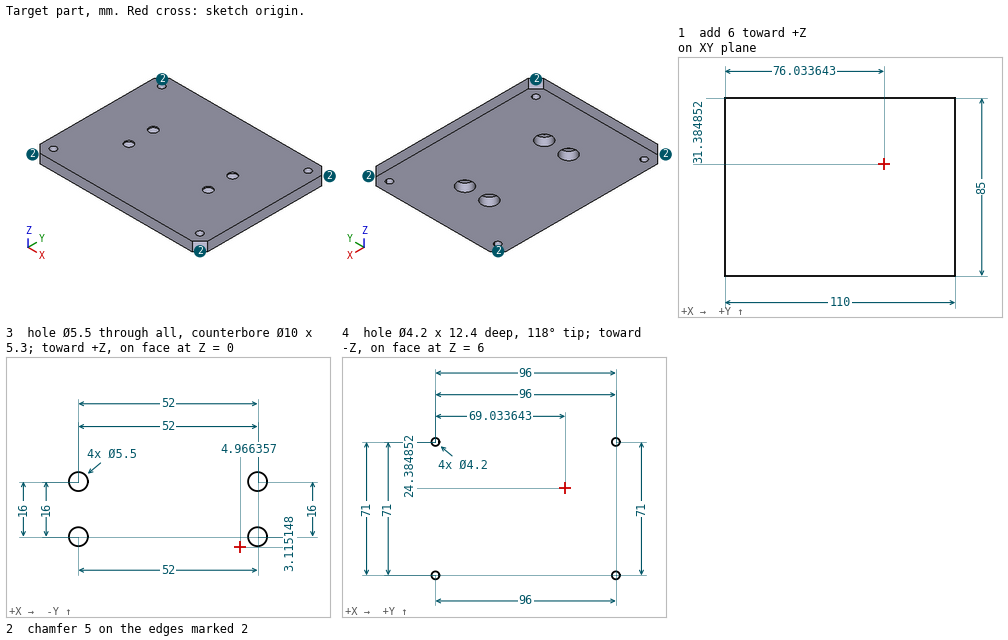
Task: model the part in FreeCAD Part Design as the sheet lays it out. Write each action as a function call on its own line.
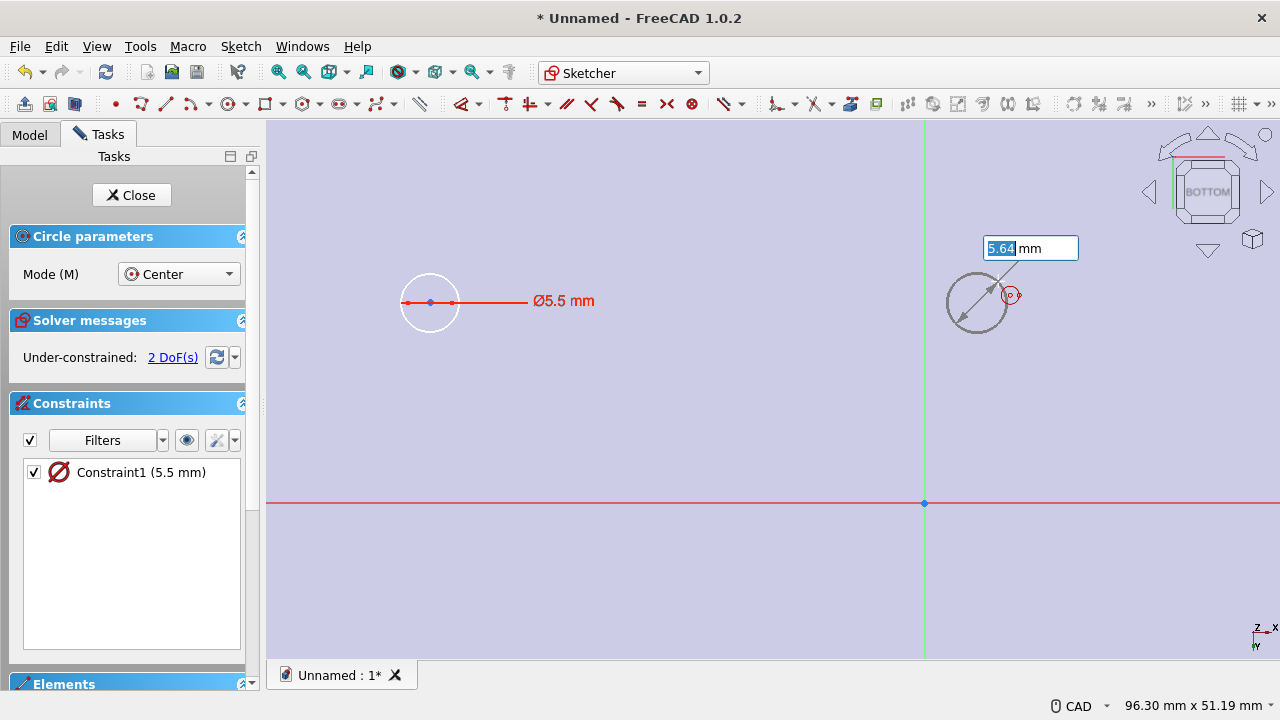
text(5.5)
key(Return)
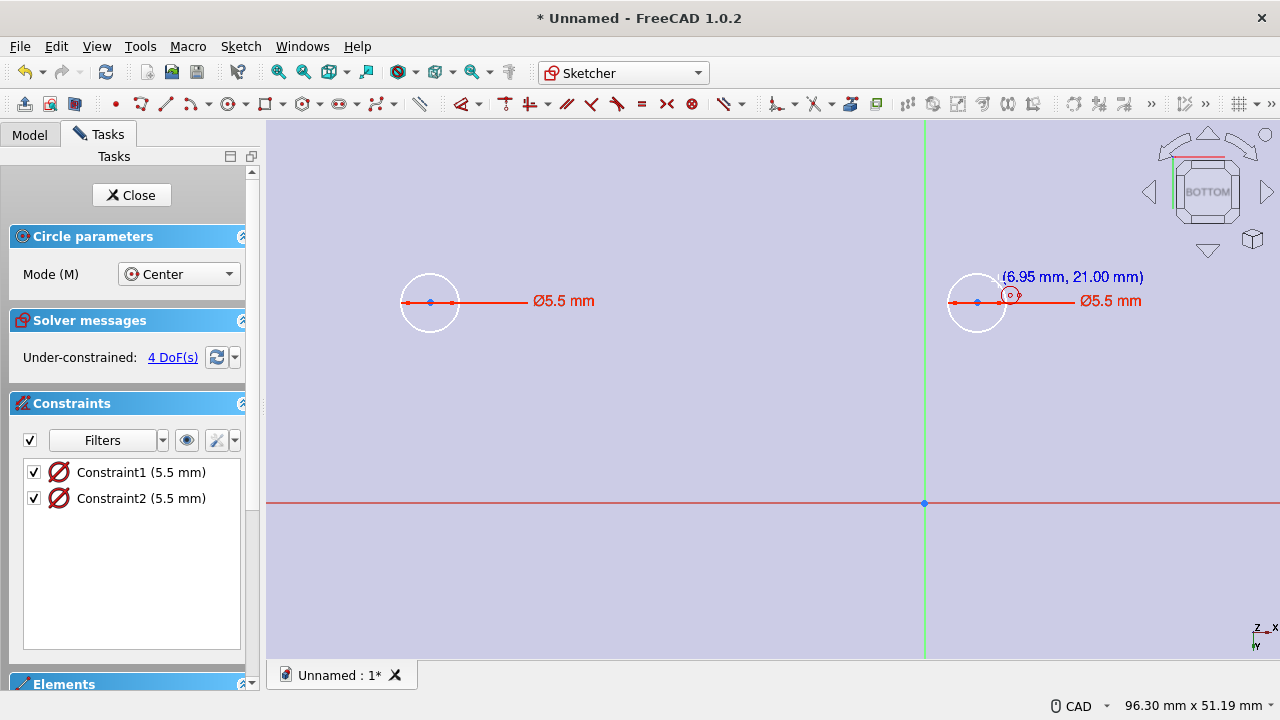
click(977, 470)
move(998, 450)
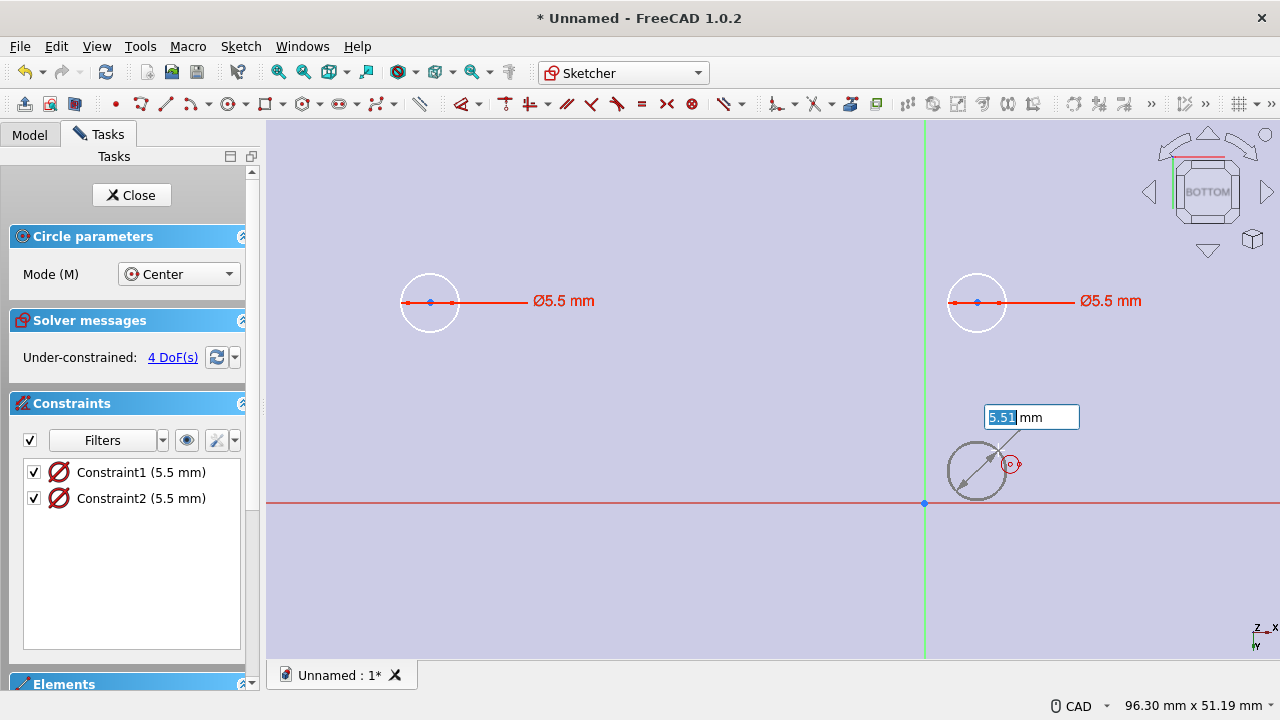
text(5.5)
key(Return)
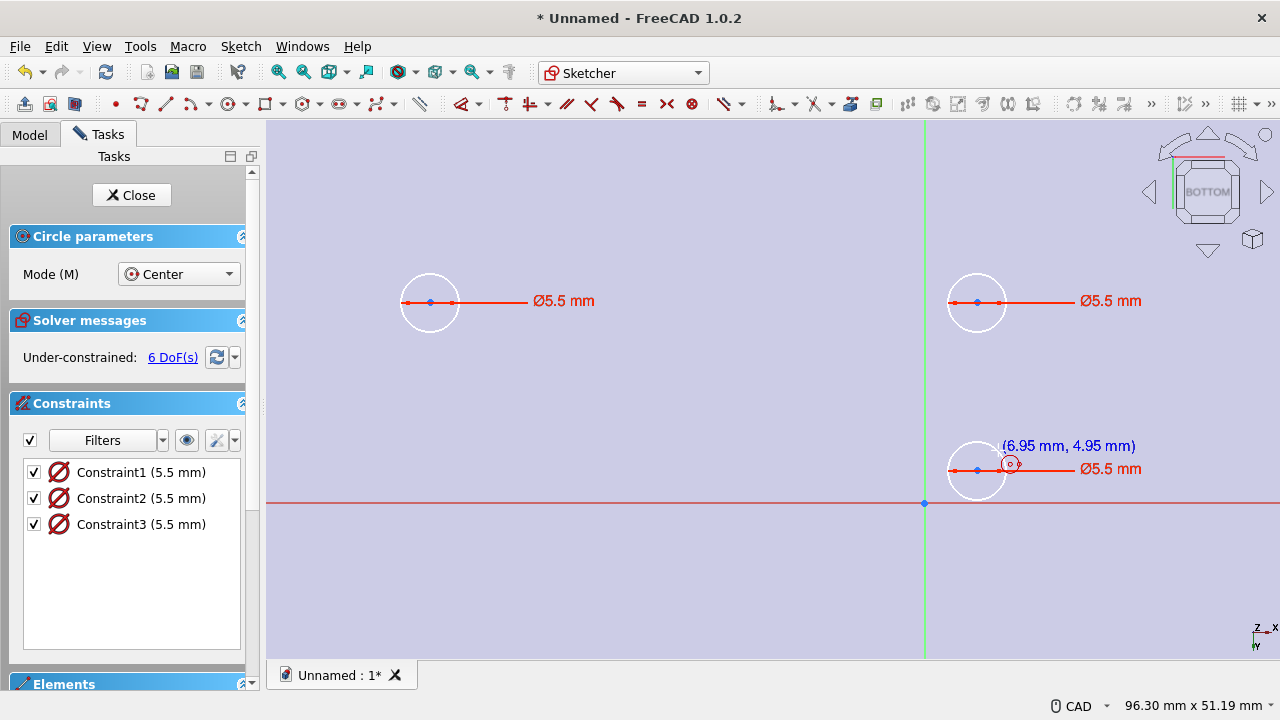
click(430, 470)
move(450, 450)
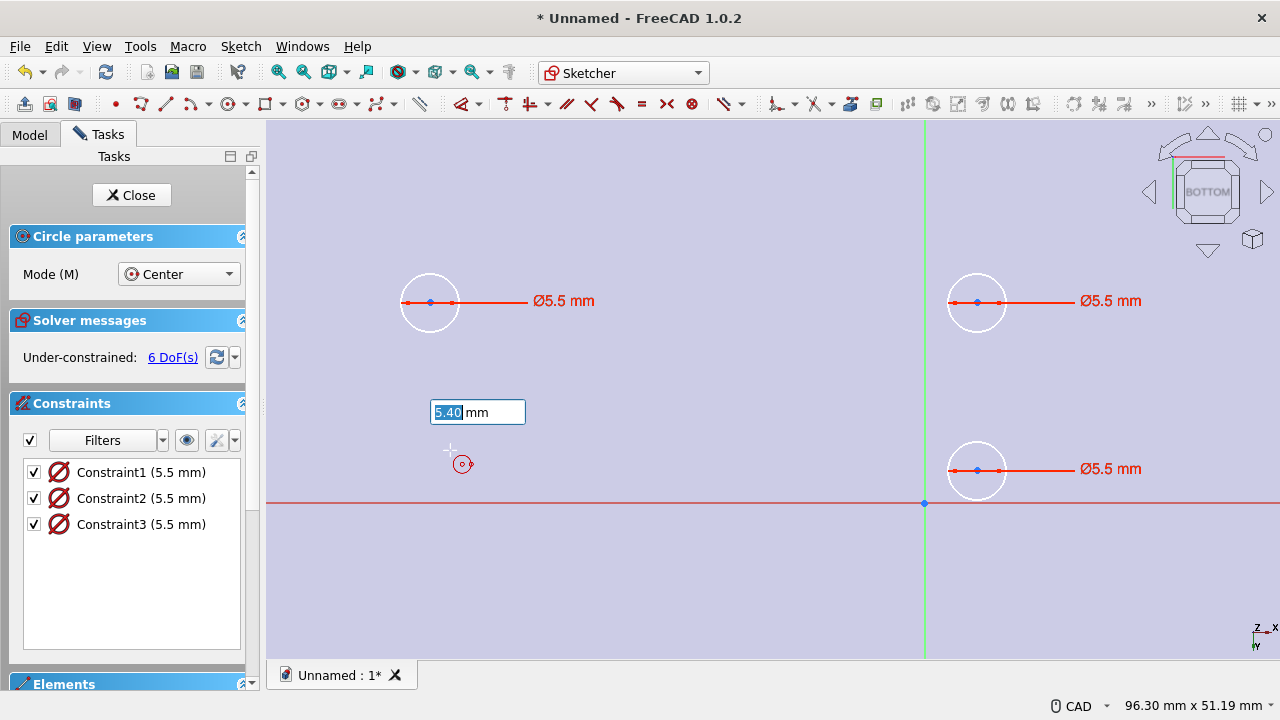
text(5.5)
key(Return)
key(Escape)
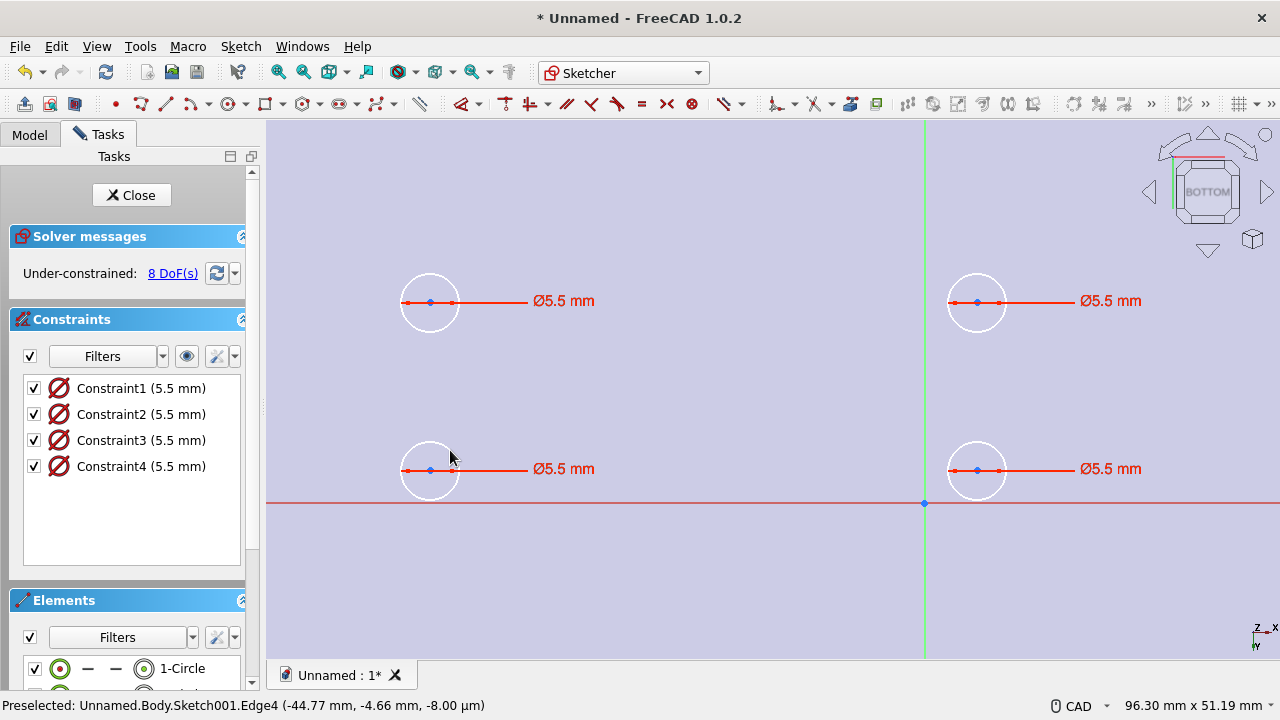
click(430, 303)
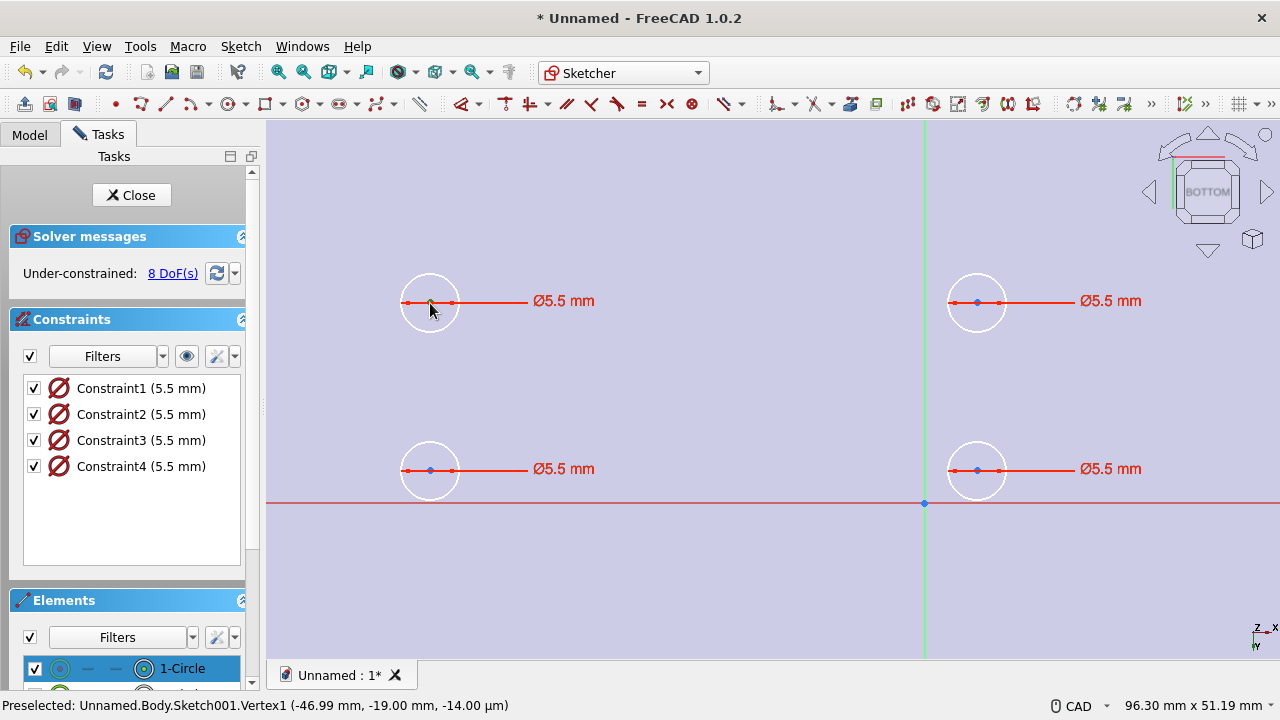
click(977, 303)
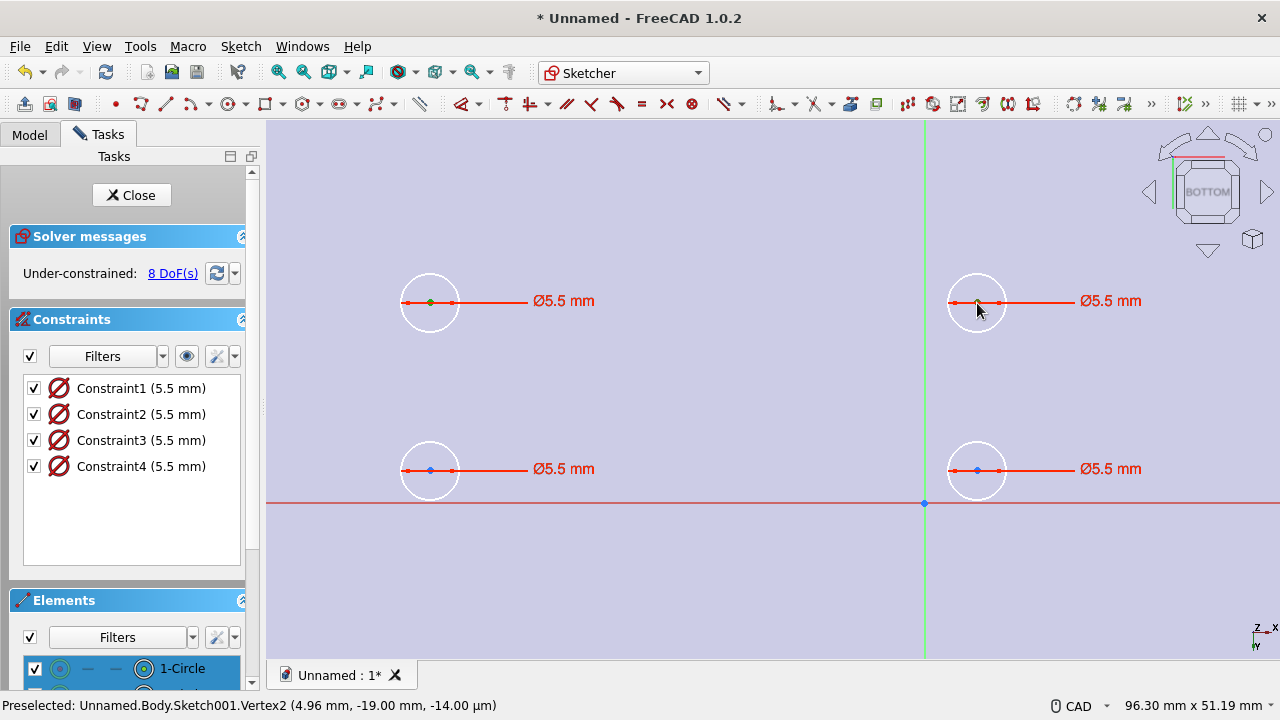
key(l)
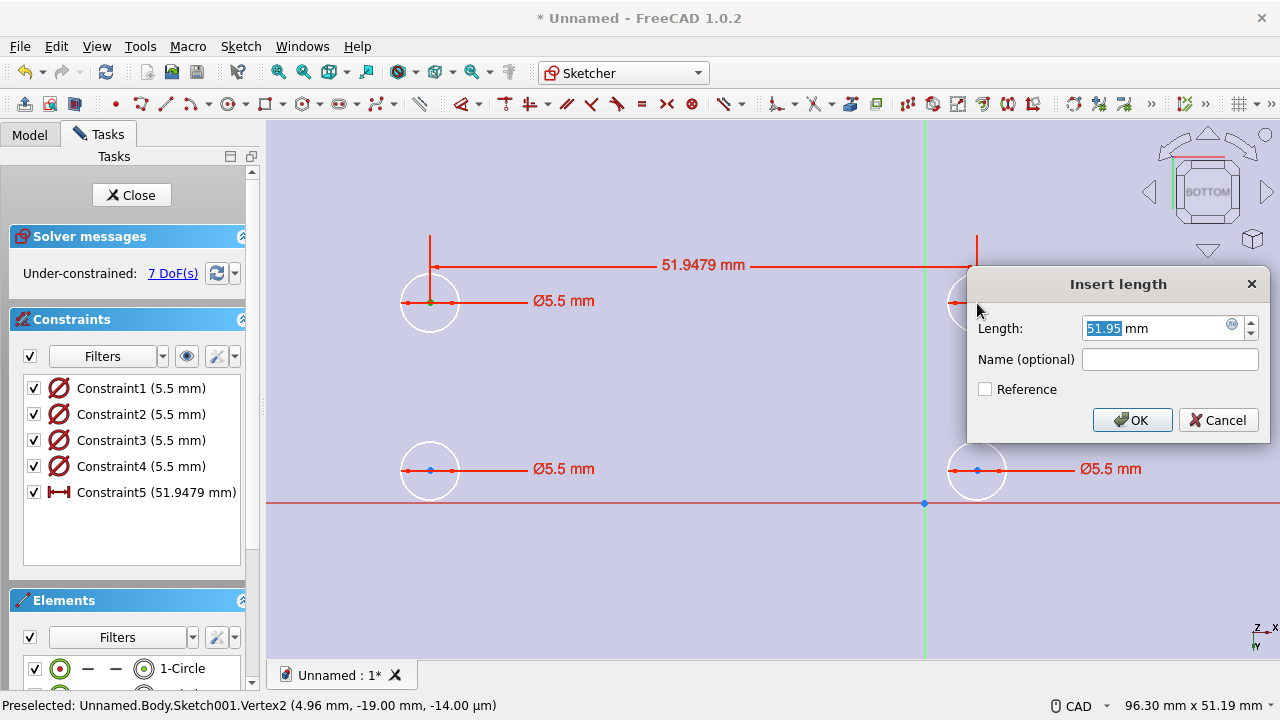
text(52)
key(Return)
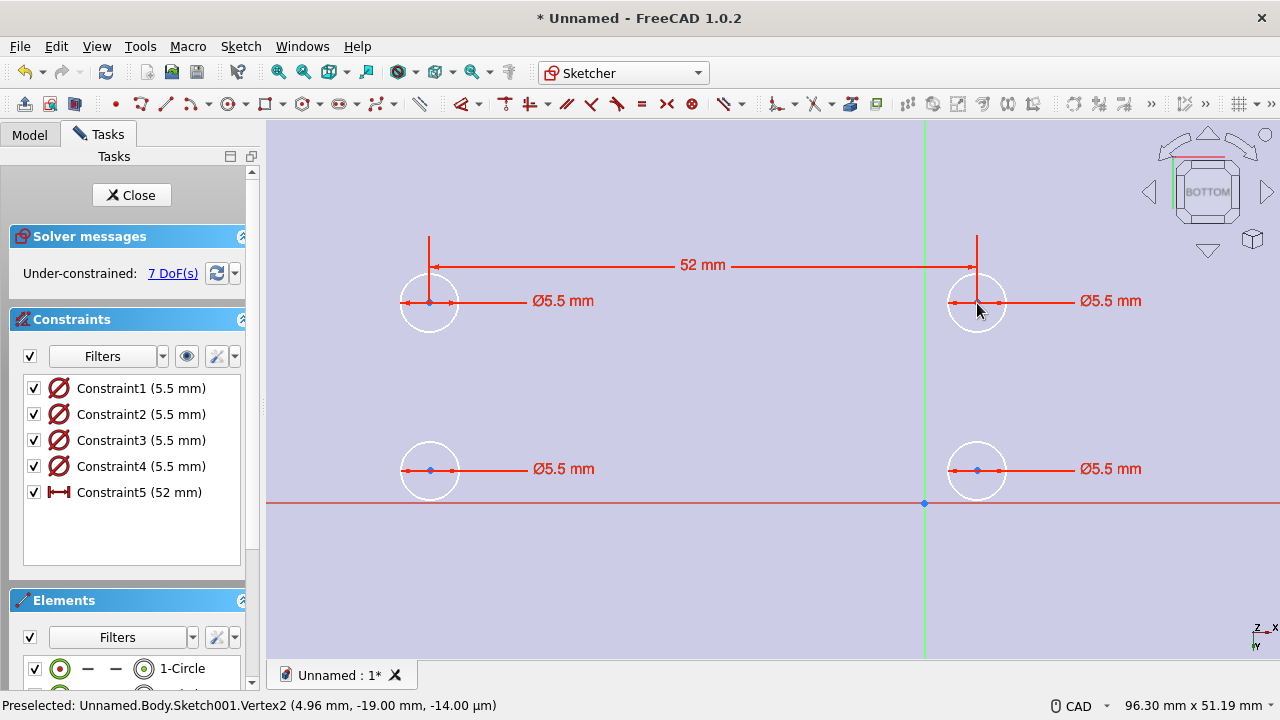
click(429, 303)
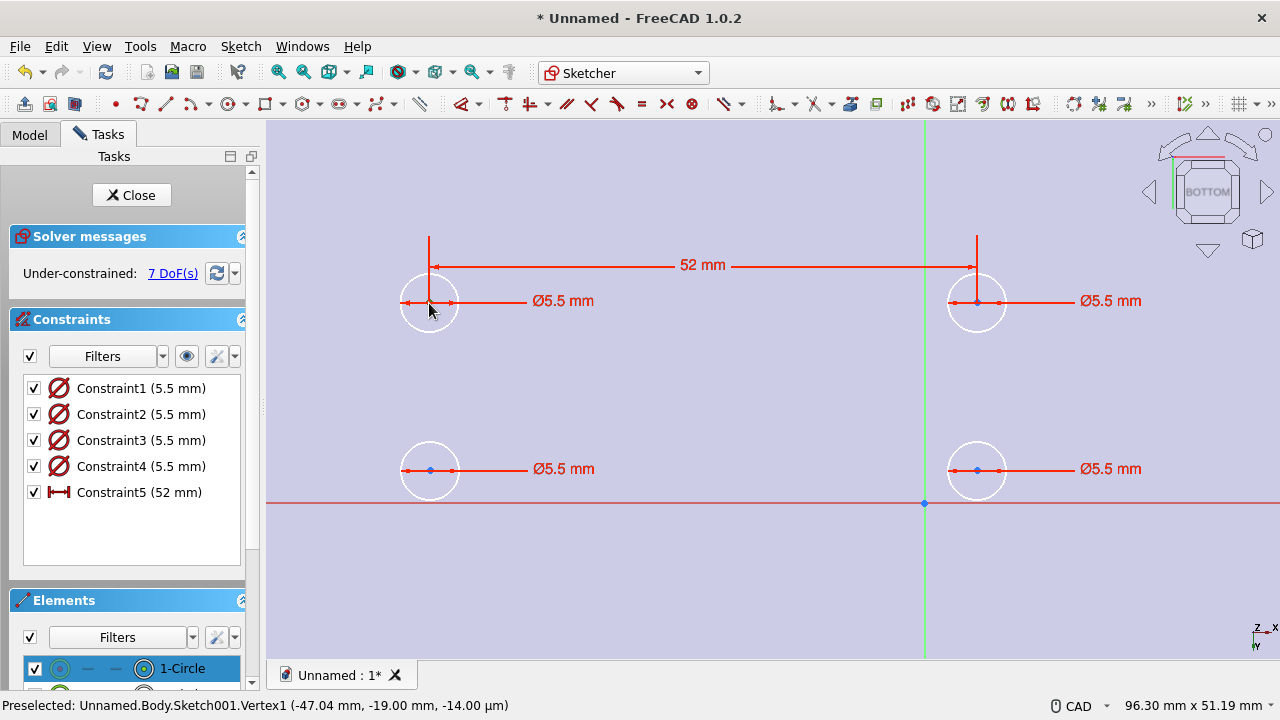
click(977, 471)